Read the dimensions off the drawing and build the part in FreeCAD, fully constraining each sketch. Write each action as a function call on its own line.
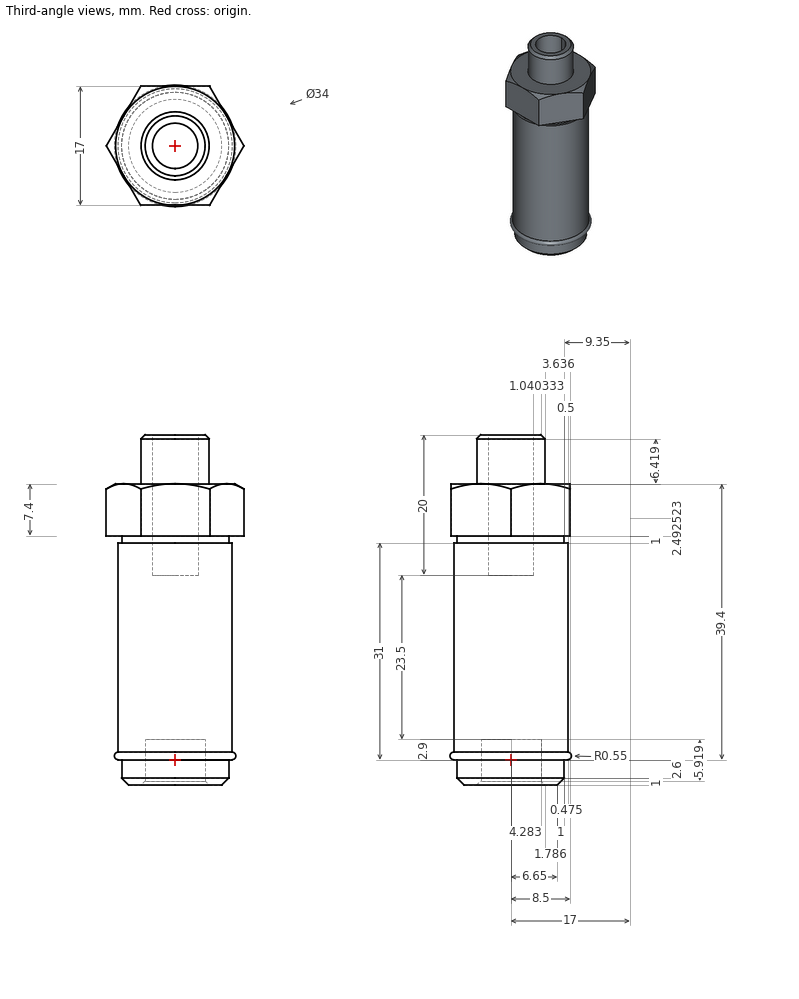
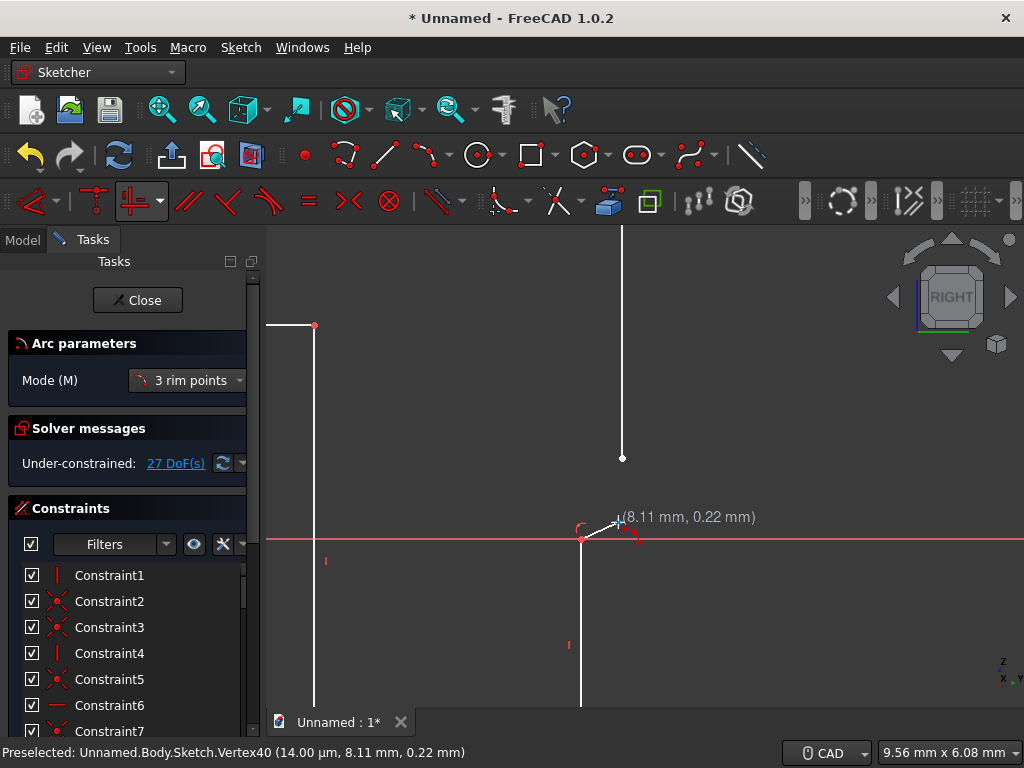
scroll(571, 596, down, 13)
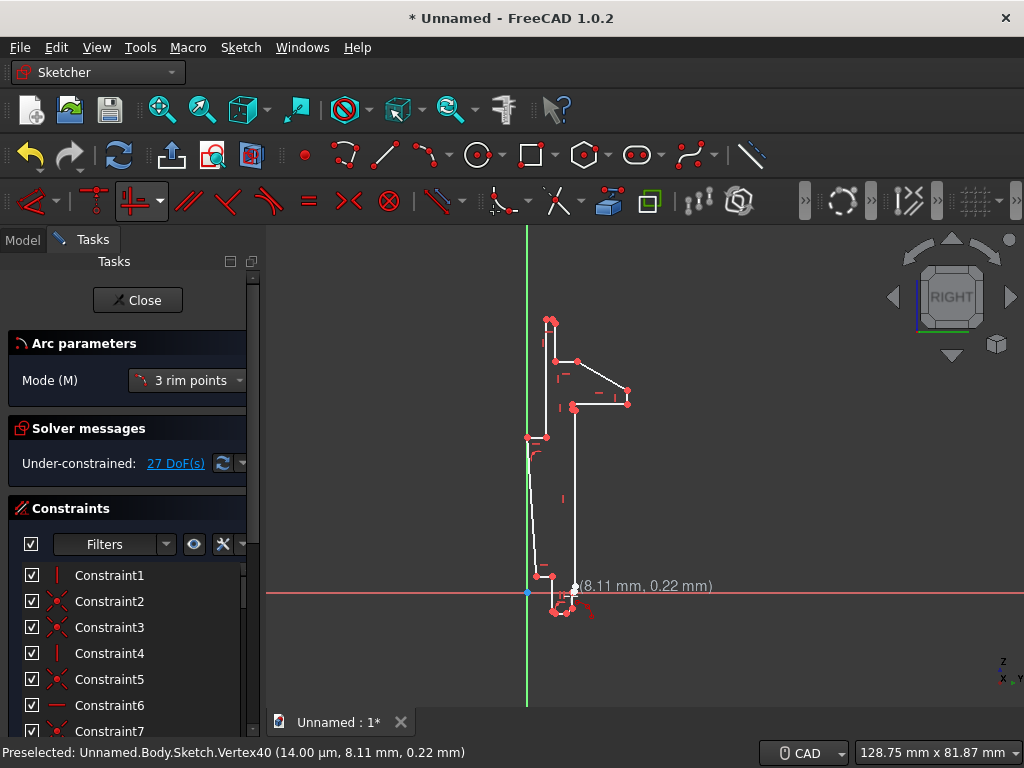
scroll(575, 586, up, 5)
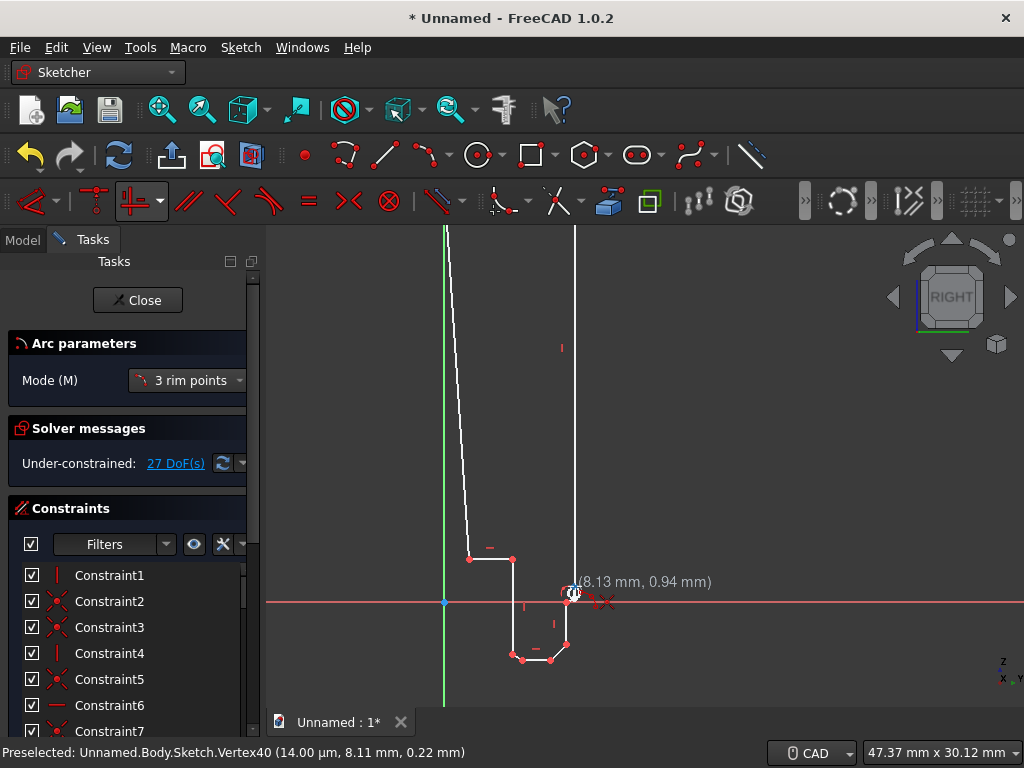
click(575, 586)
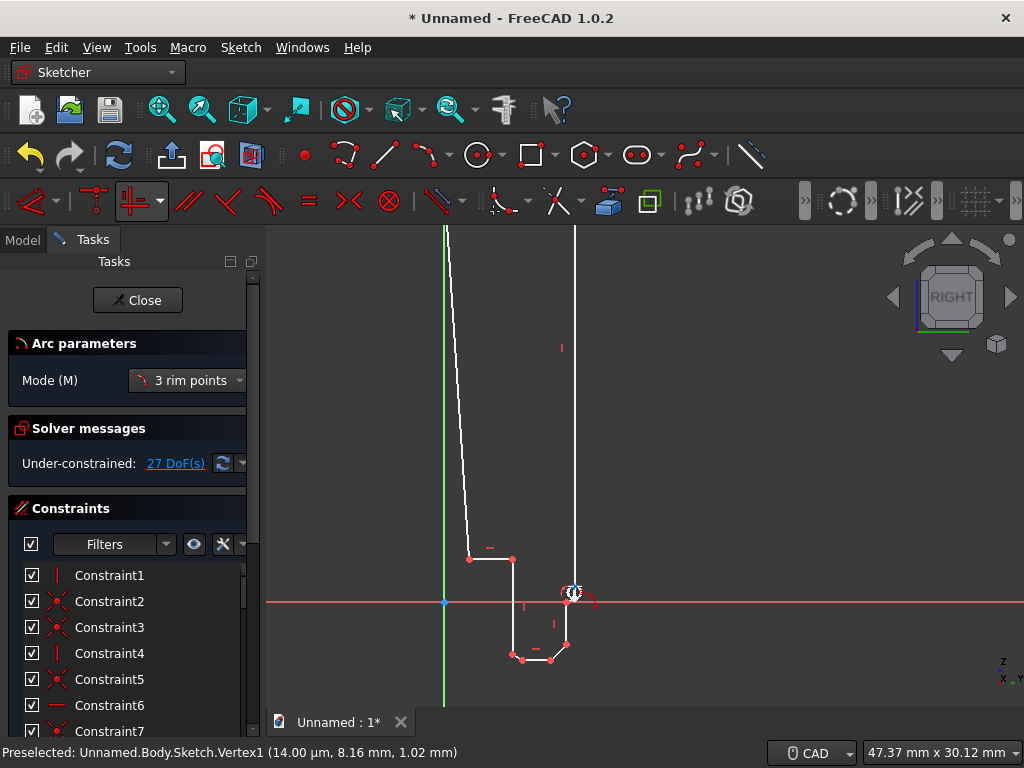
scroll(583, 594, up, 4)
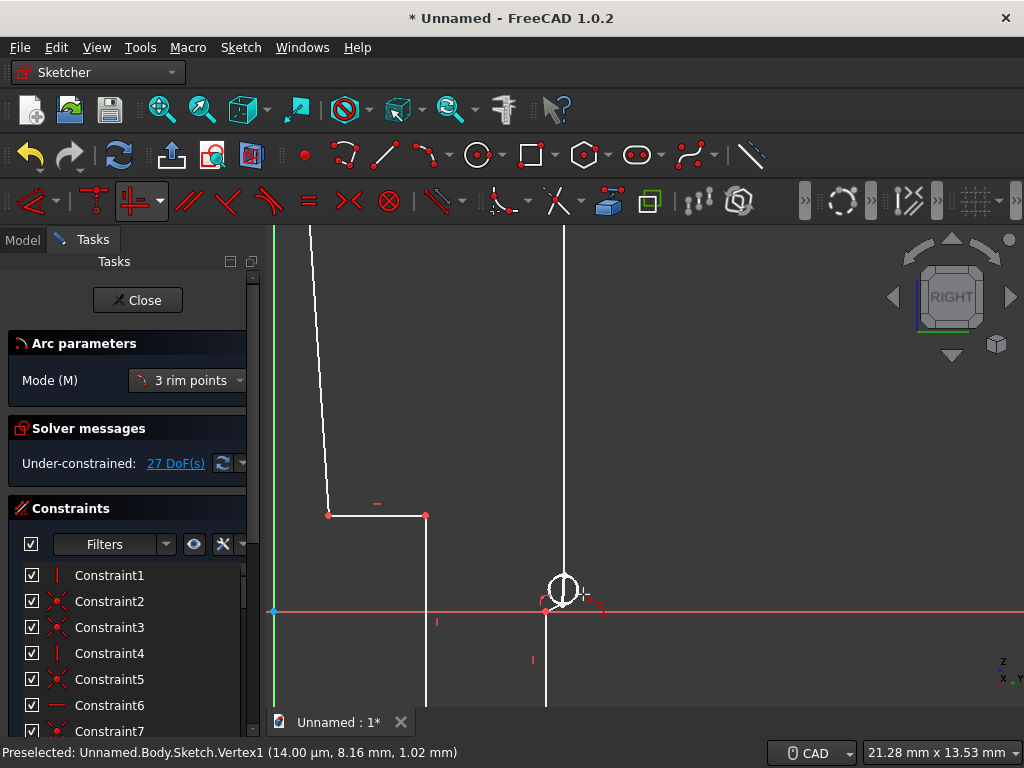
click(582, 593)
key(Escape)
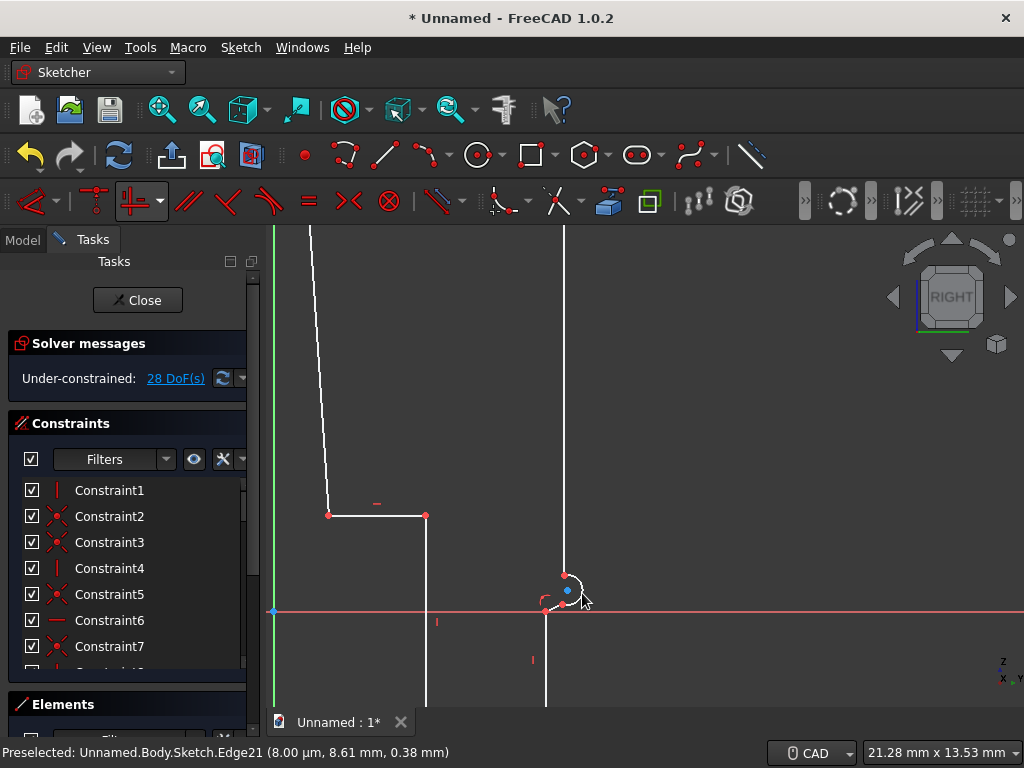
scroll(554, 608, up, 3)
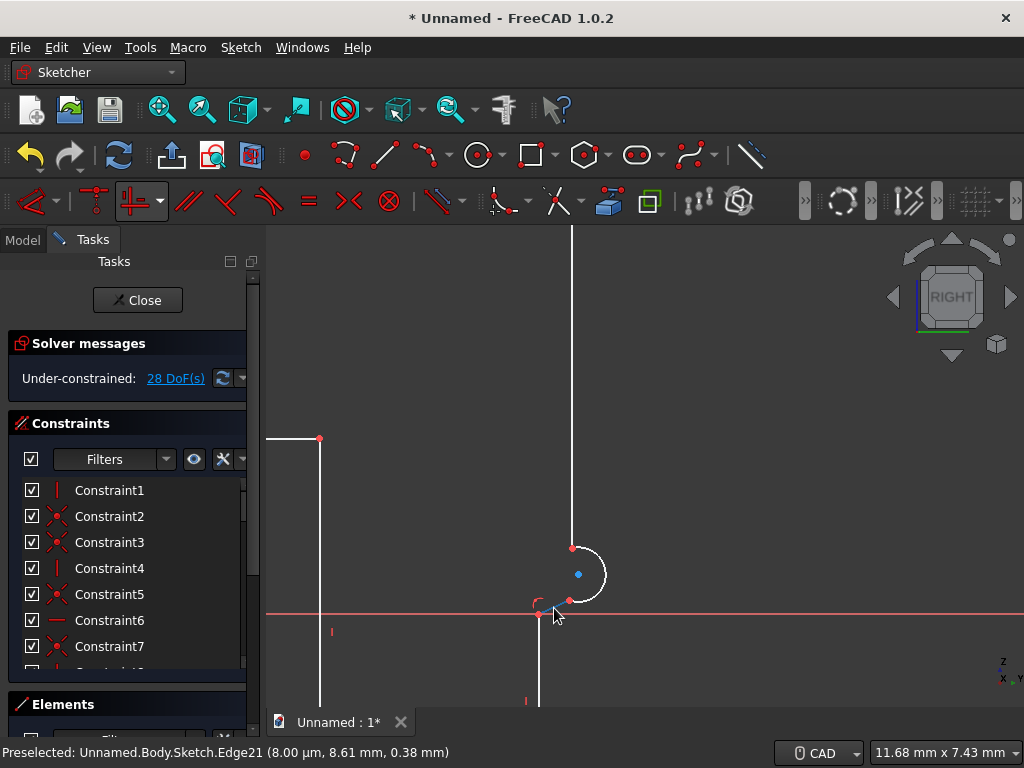
click(554, 607)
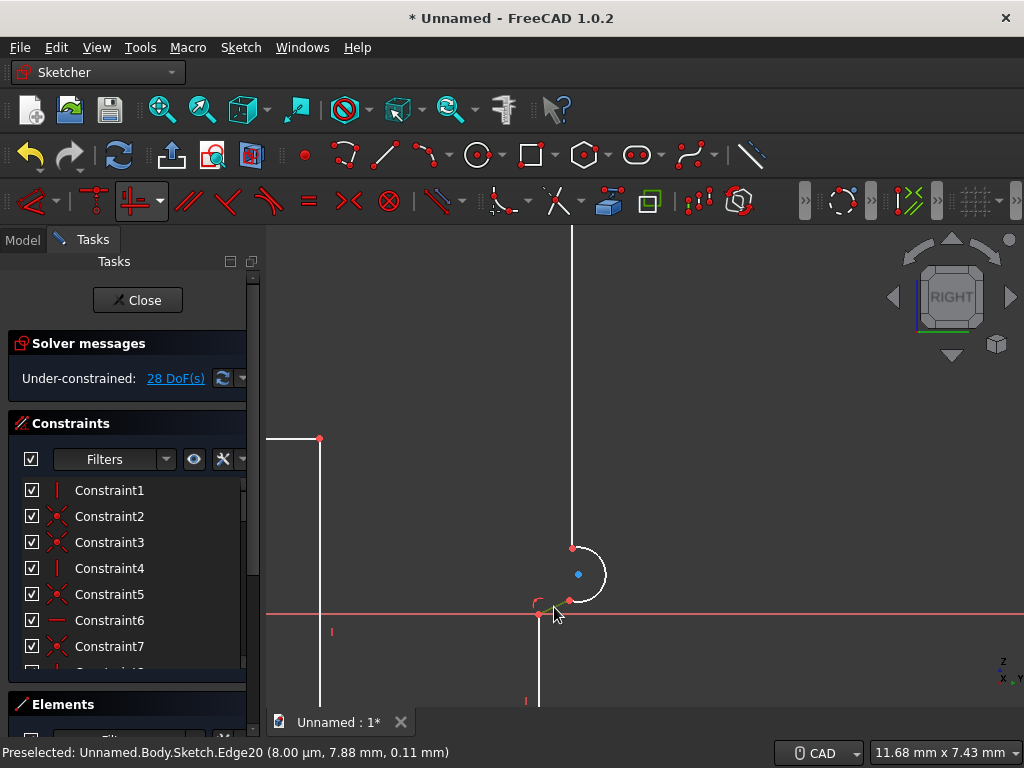
click(597, 594)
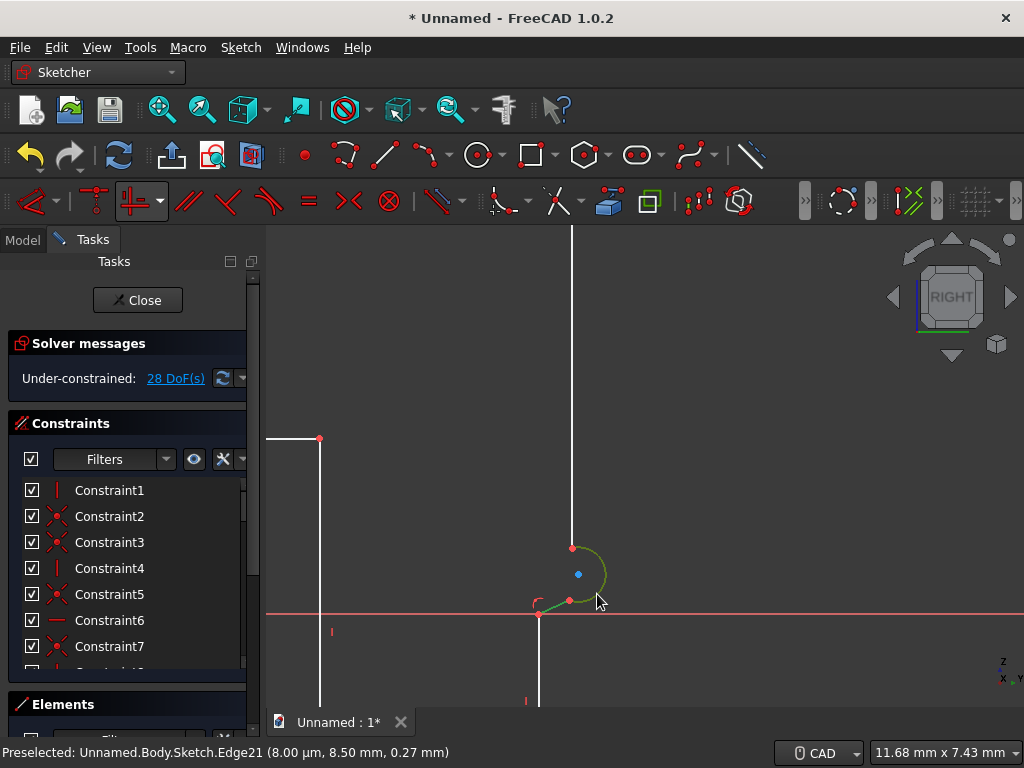
key(t)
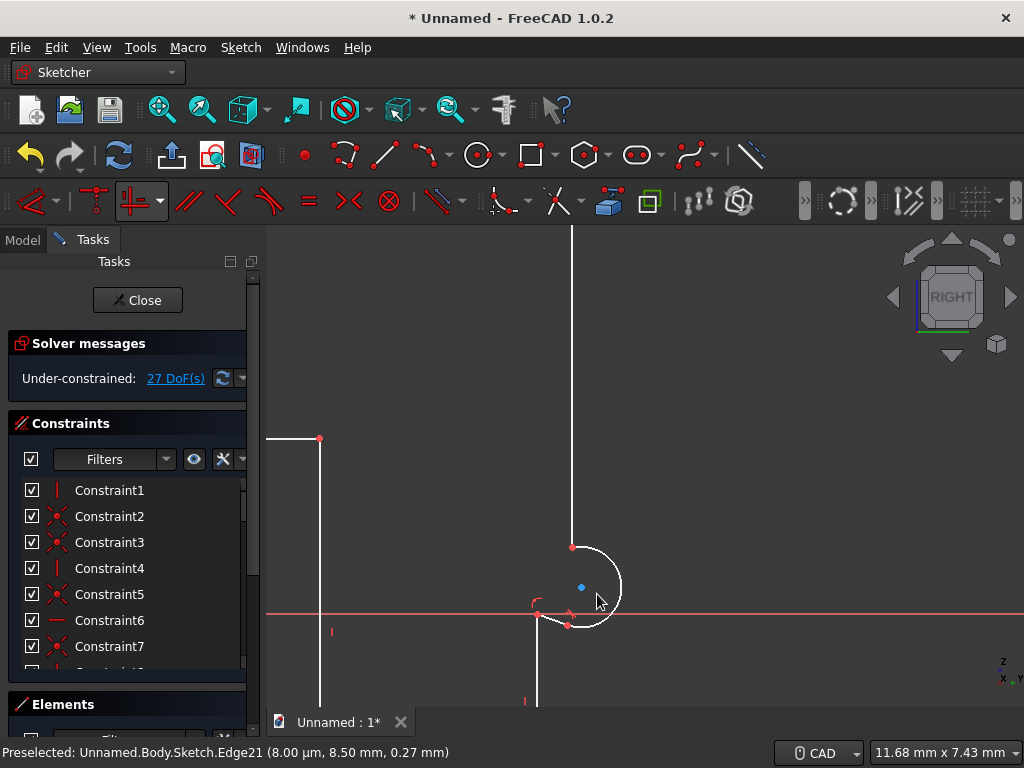
scroll(575, 590, down, 12)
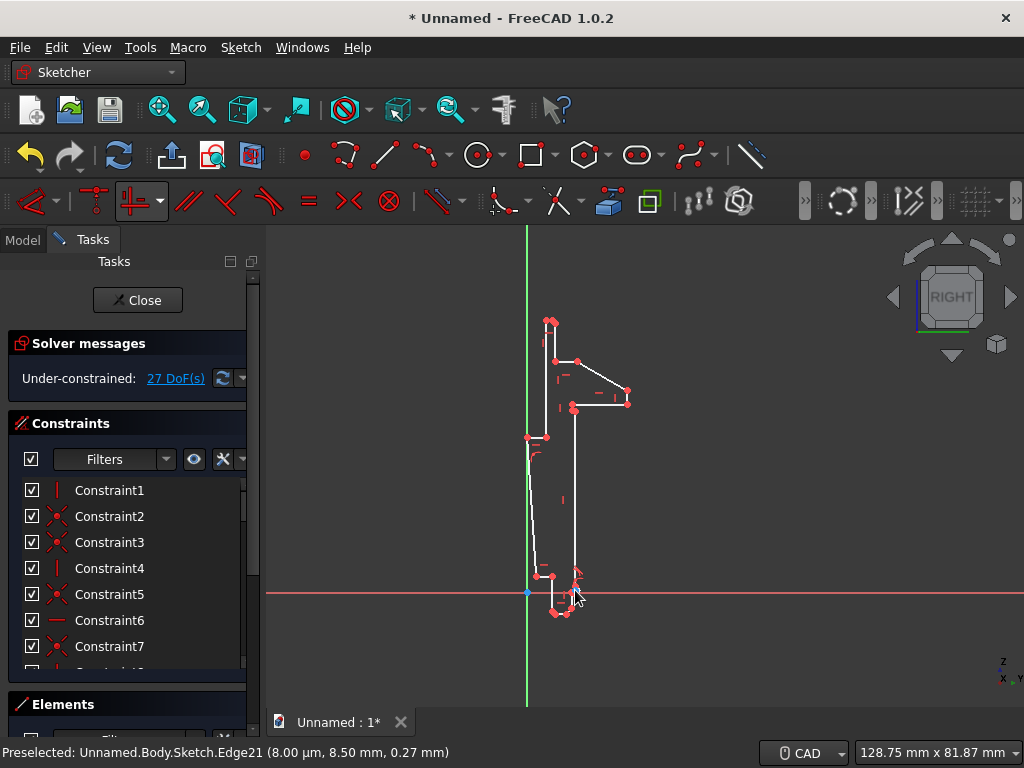
scroll(574, 411, up, 14)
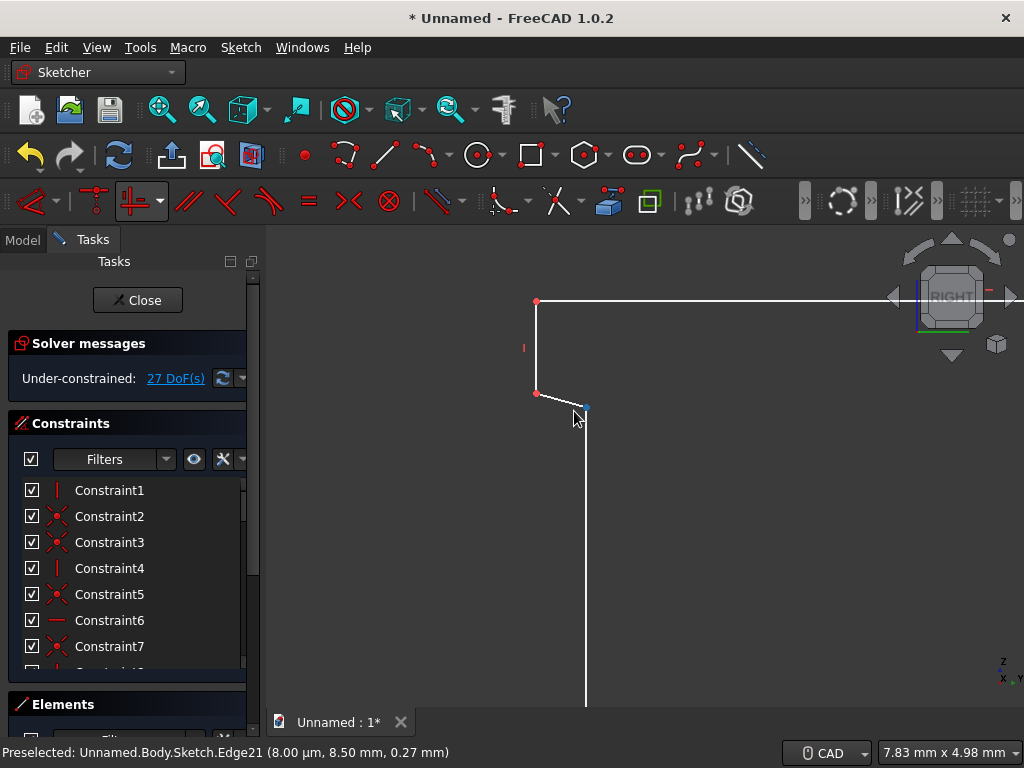
click(571, 403)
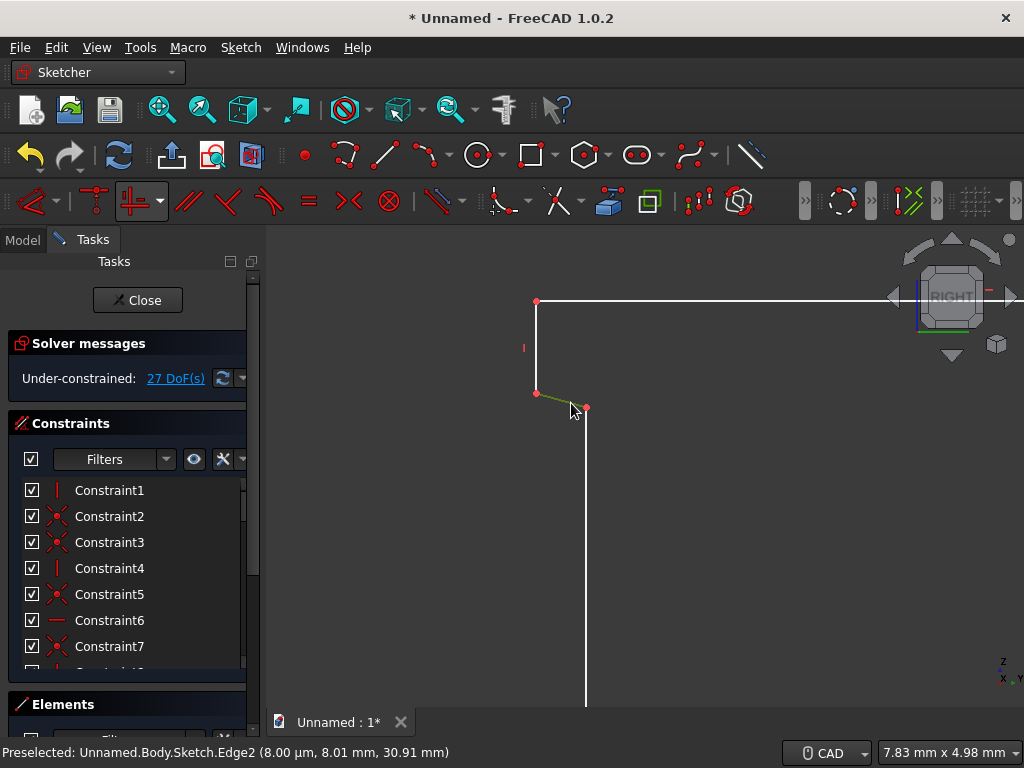
key(h)